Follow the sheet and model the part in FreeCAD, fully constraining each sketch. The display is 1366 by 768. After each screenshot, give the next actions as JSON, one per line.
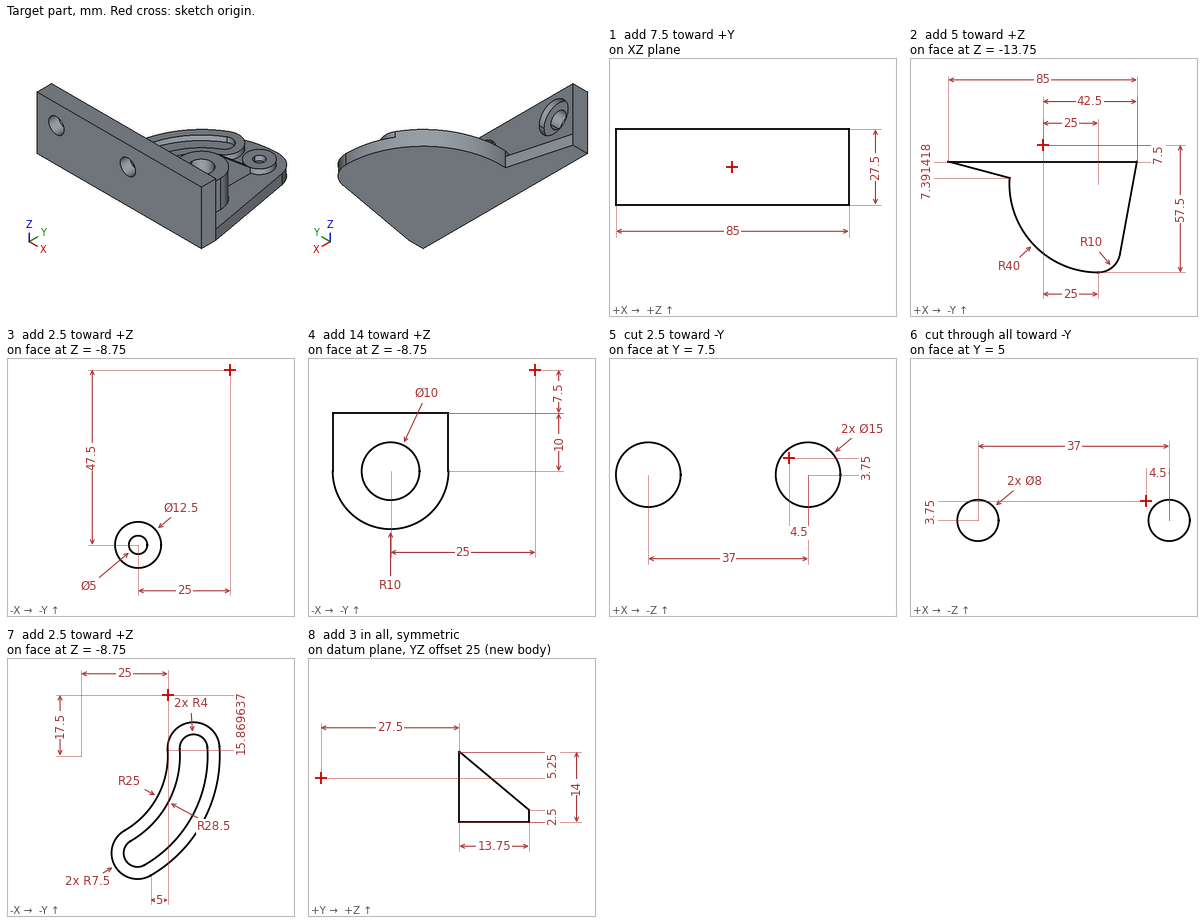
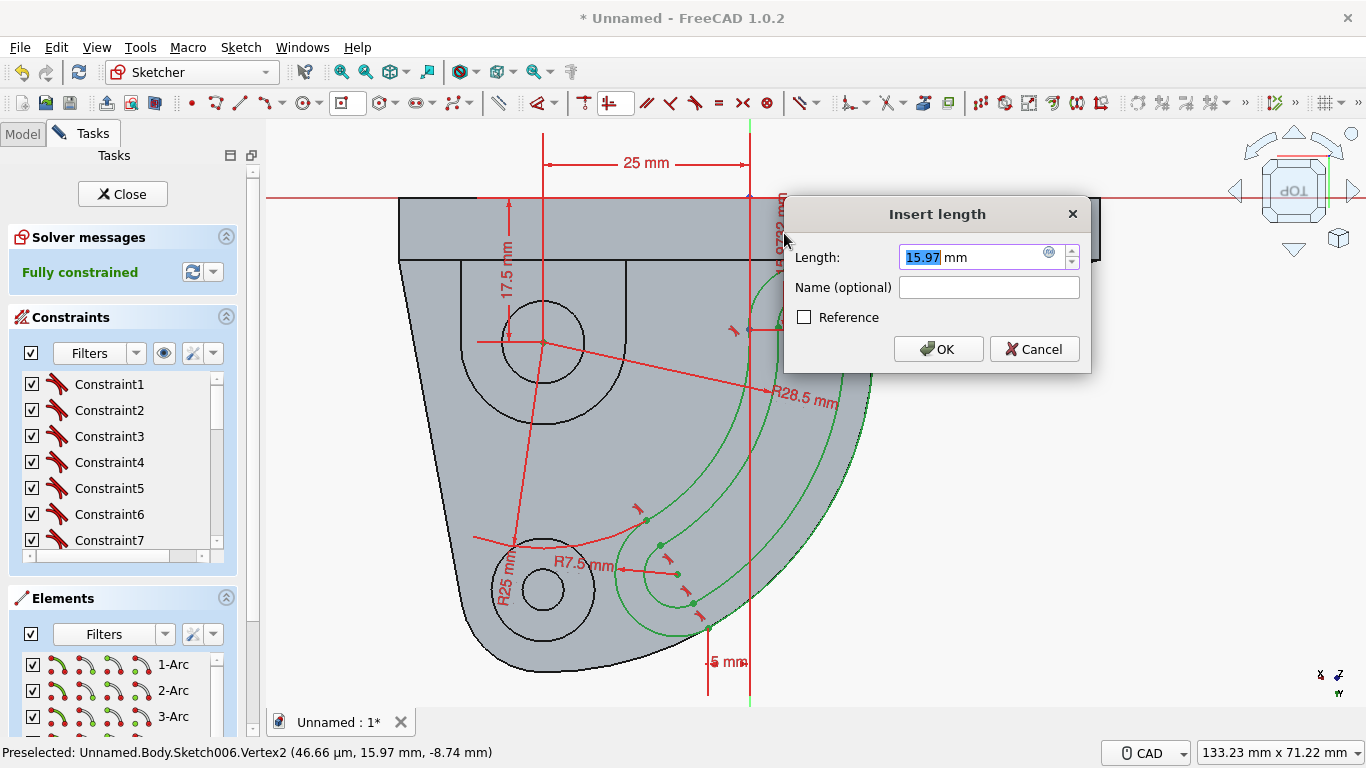
{"action": "type", "text": "15.869637"}
{"action": "key", "text": "Return"}
{"action": "key", "text": "Escape"}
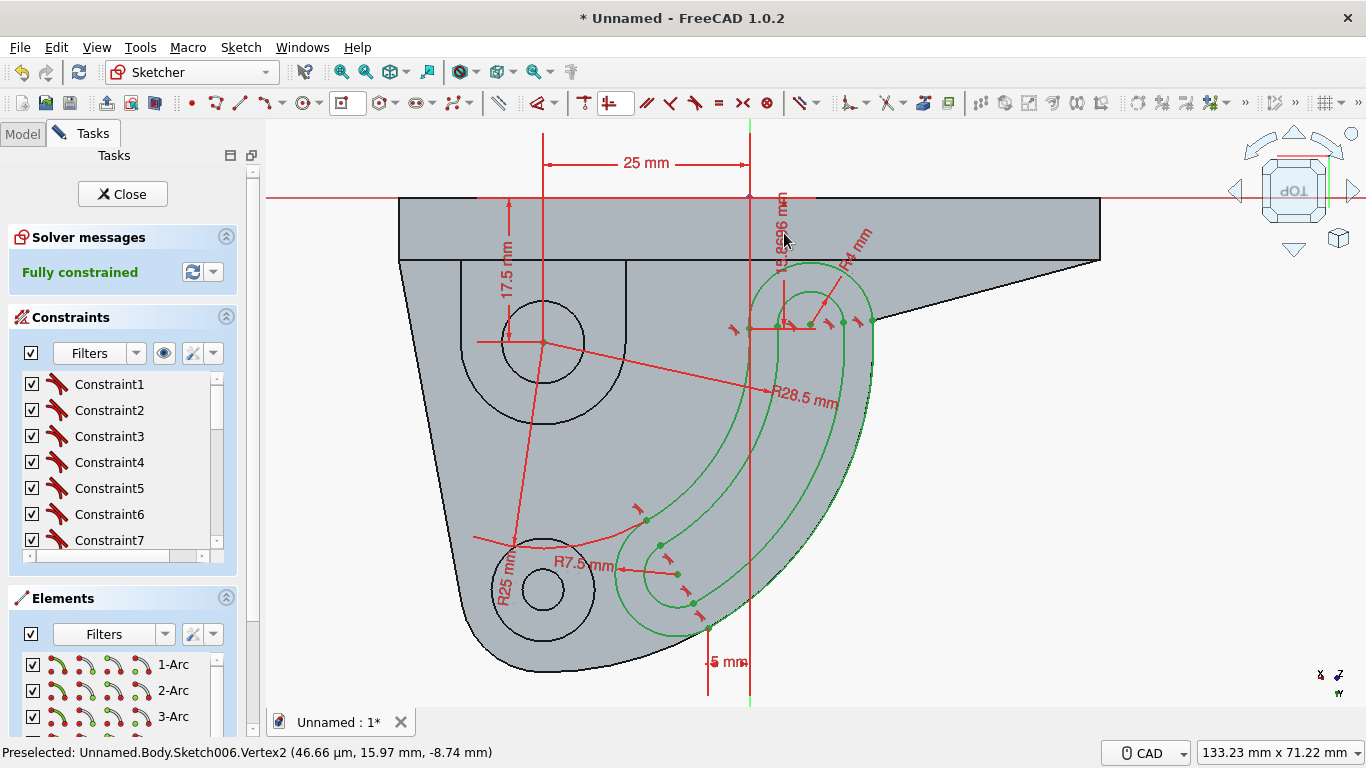
{"action": "left_click", "coordinate": [123, 194]}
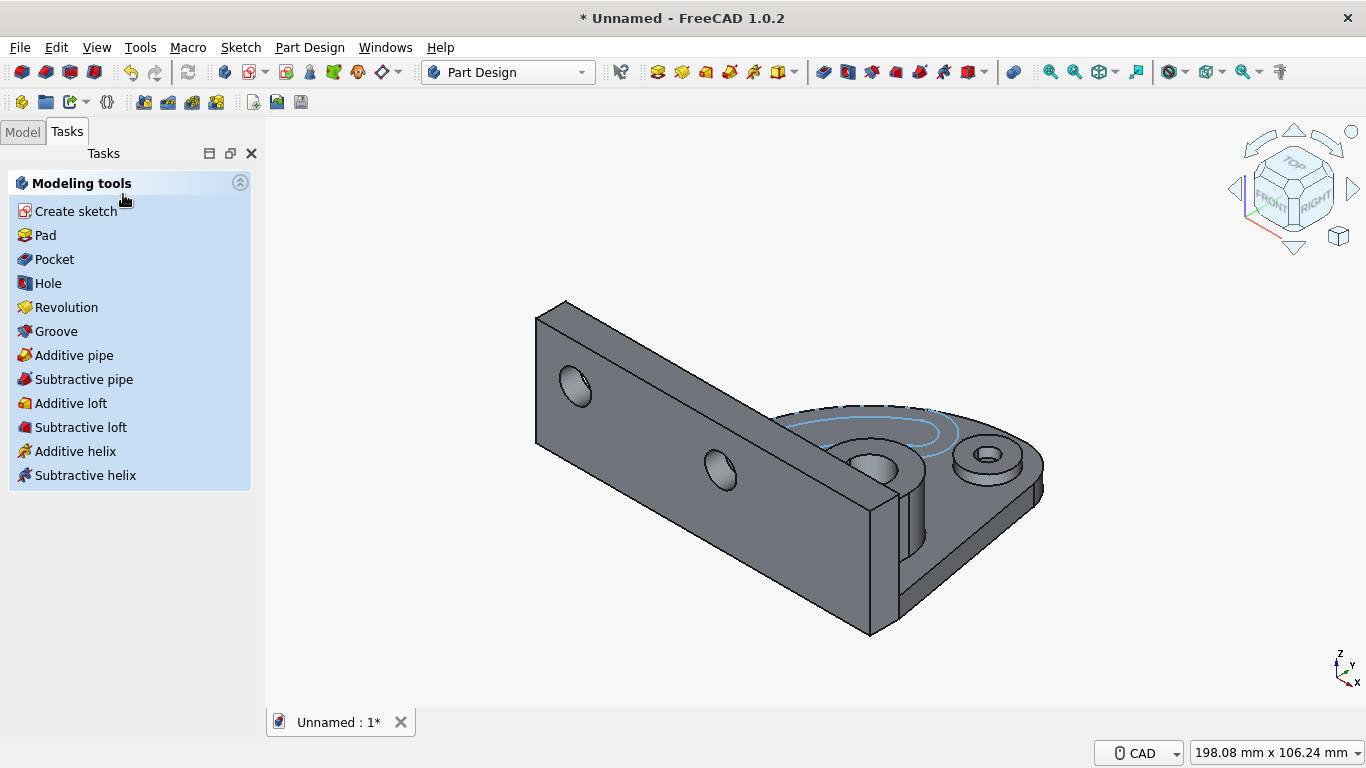
{"action": "left_click", "coordinate": [658, 72]}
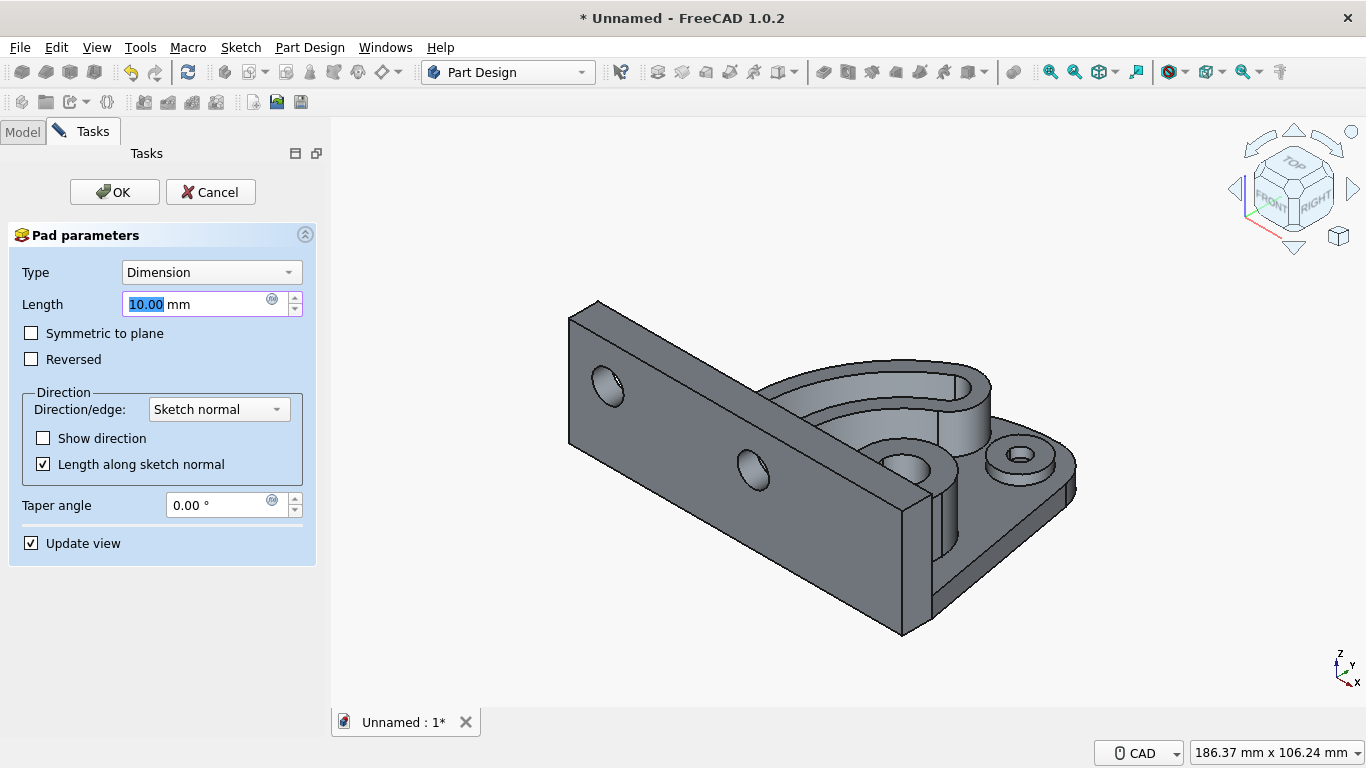
{"action": "type", "text": "2.5"}
{"action": "key", "text": "Tab"}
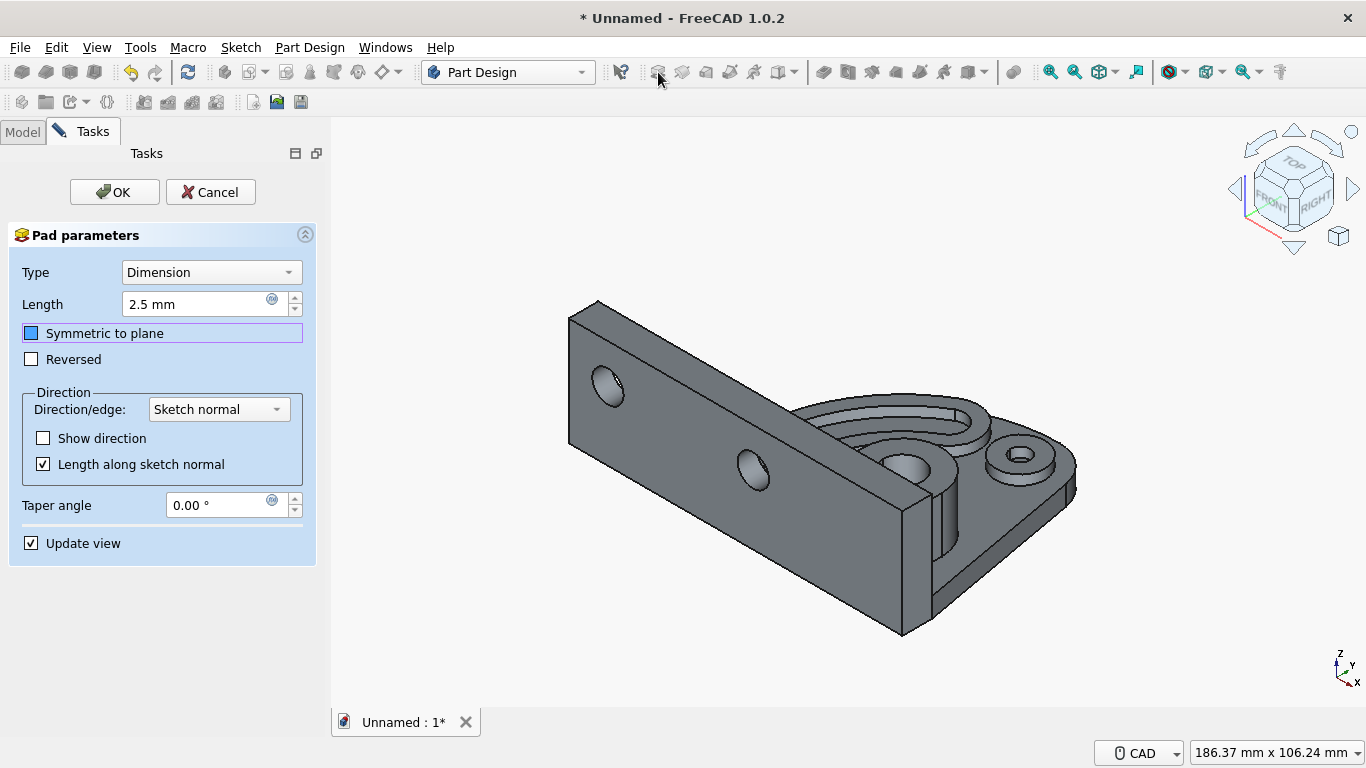
{"action": "left_click", "coordinate": [115, 192]}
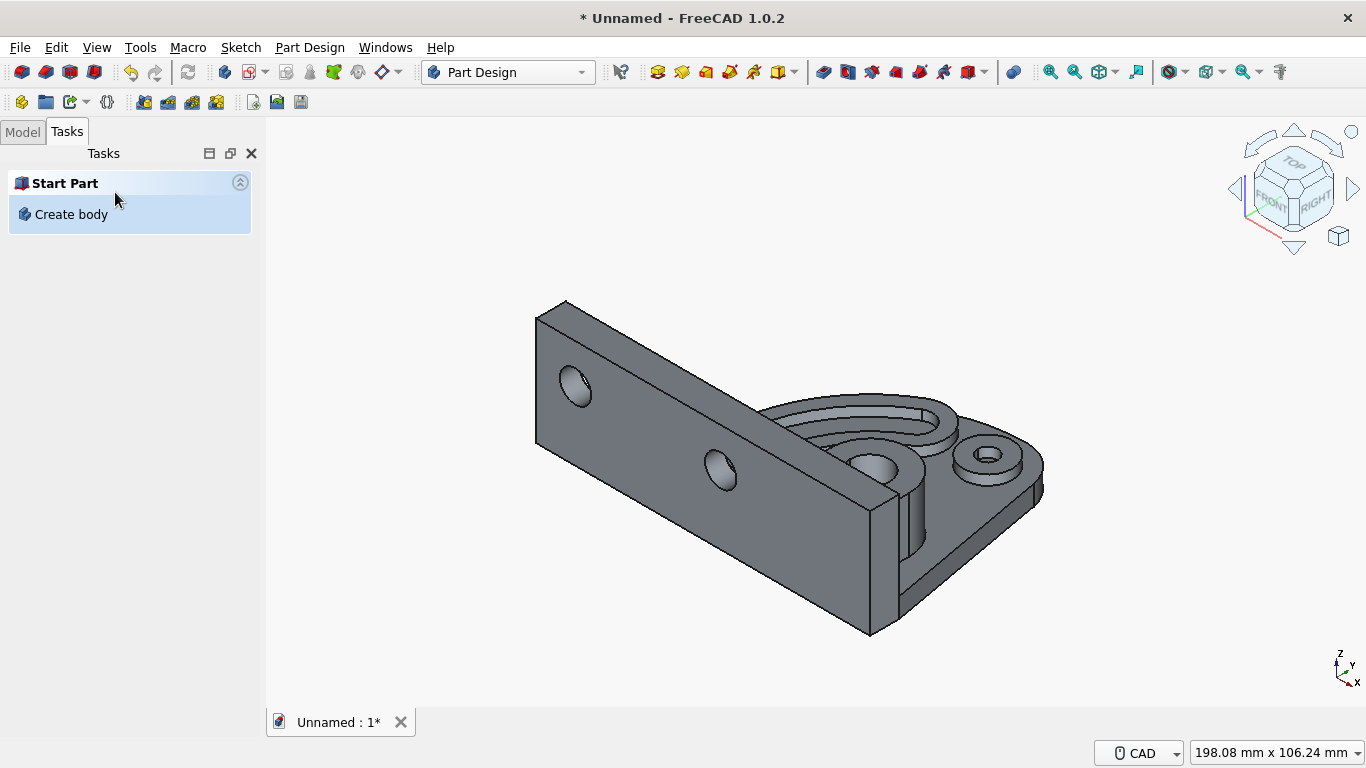
{"action": "left_click", "coordinate": [226, 72]}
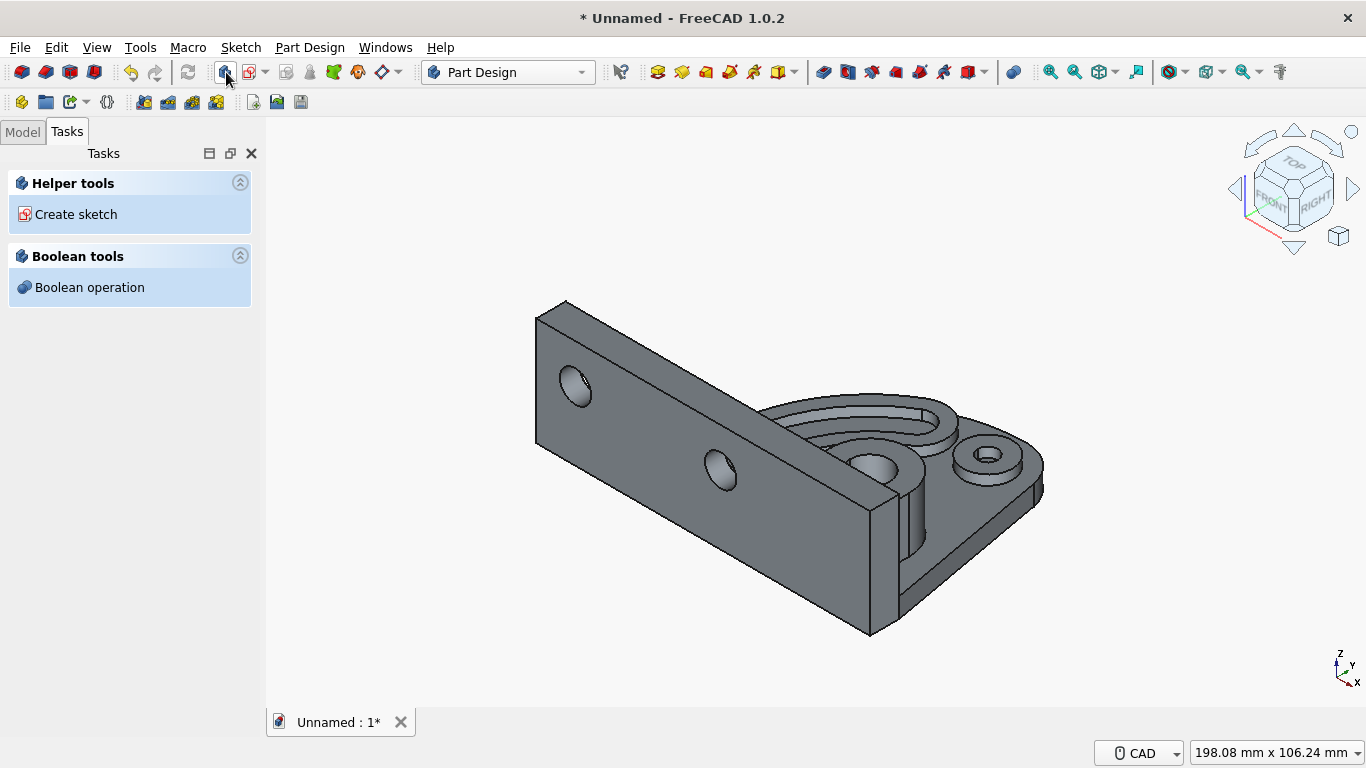
{"action": "left_click", "coordinate": [23, 131]}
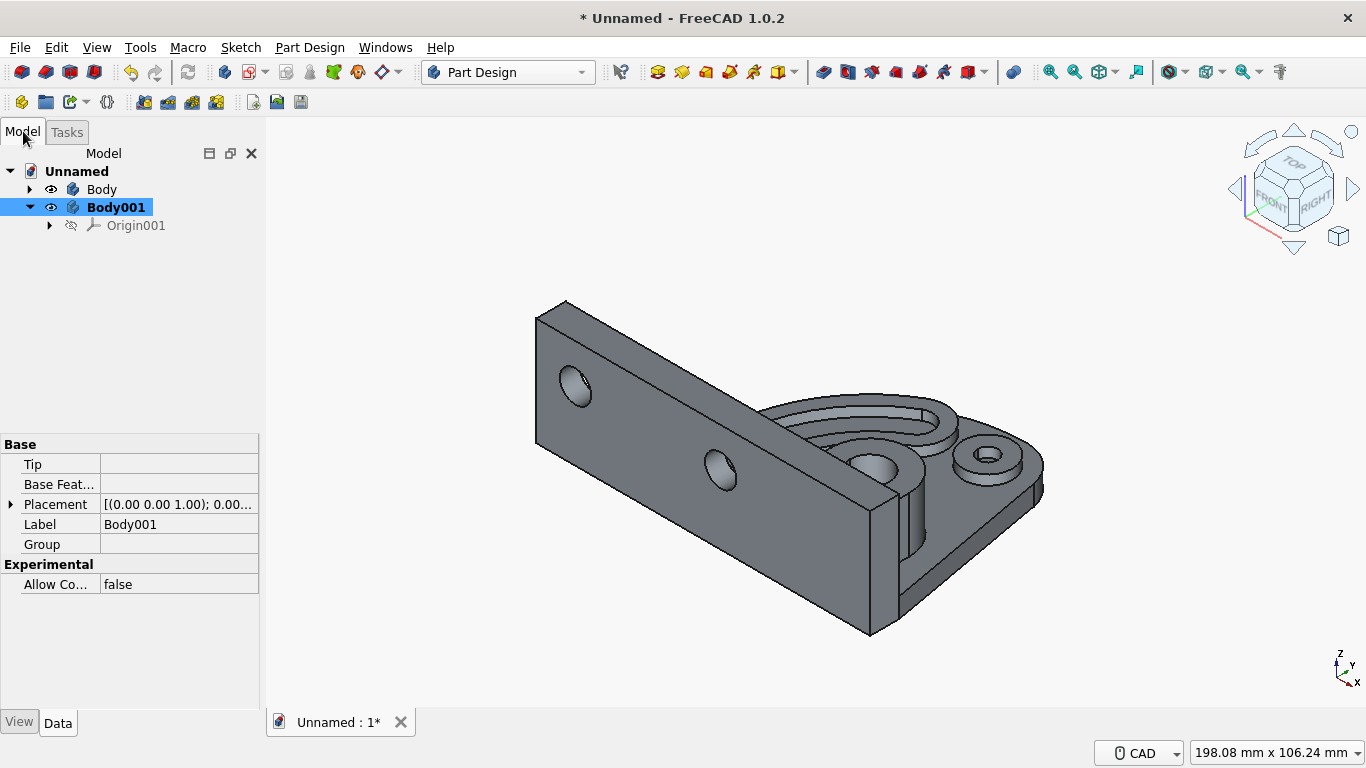
{"action": "left_click", "coordinate": [50, 225]}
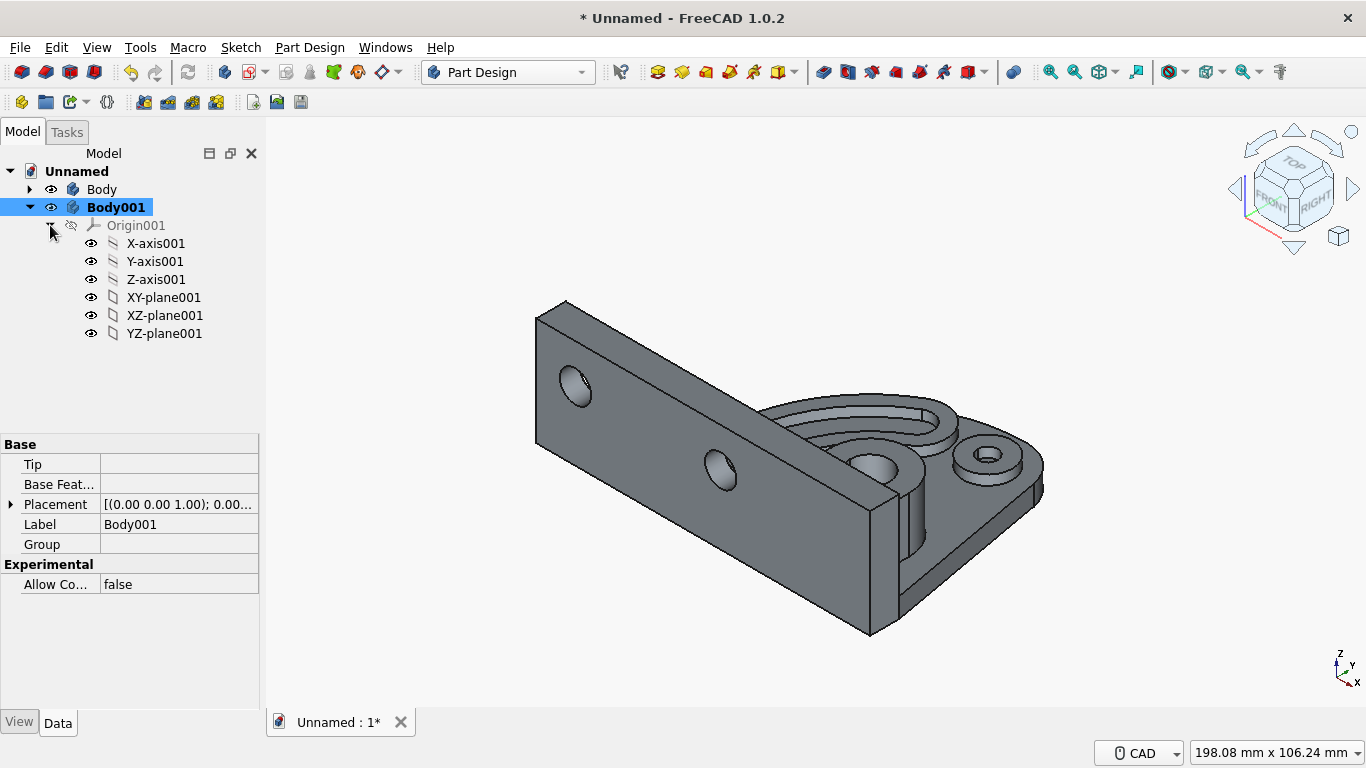
{"action": "left_click", "coordinate": [136, 333]}